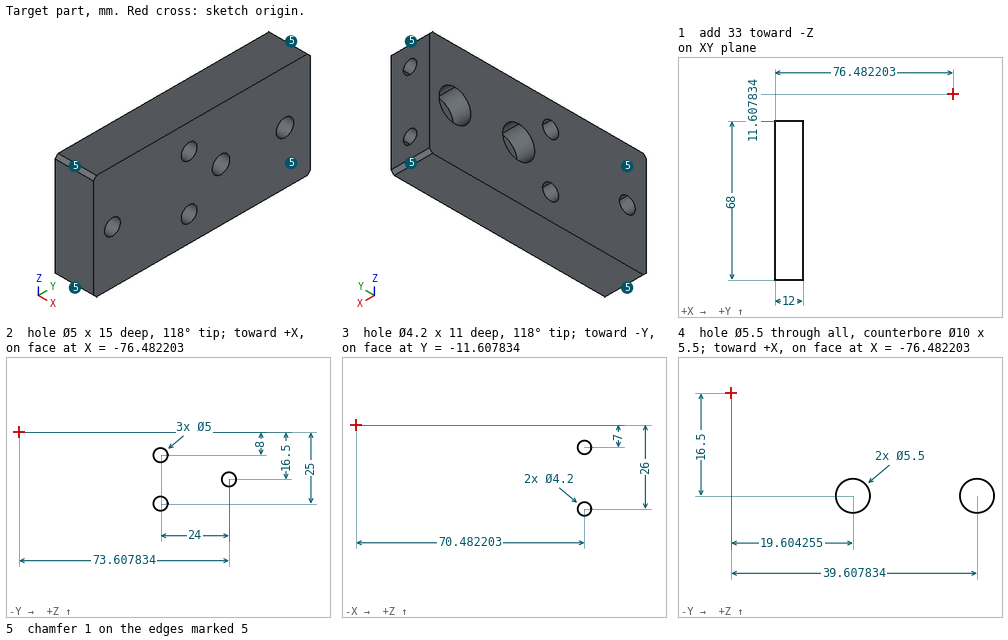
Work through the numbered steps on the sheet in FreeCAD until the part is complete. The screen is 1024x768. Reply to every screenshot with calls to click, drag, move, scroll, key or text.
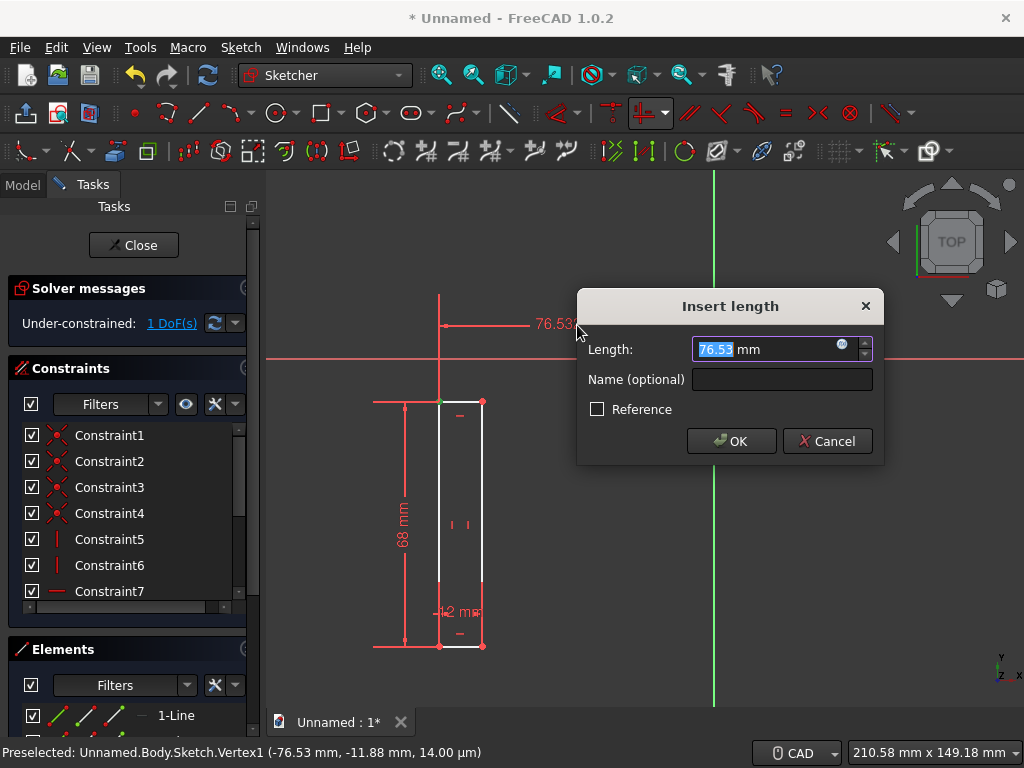
text(76.482203)
key(Return)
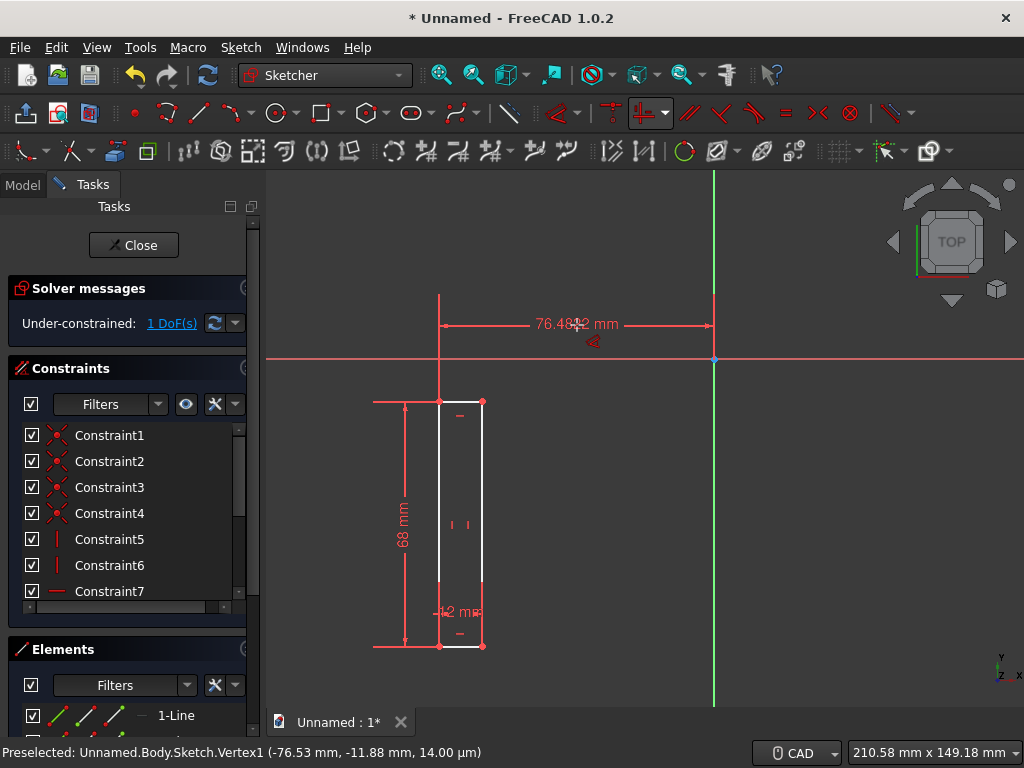
click(439, 402)
click(405, 381)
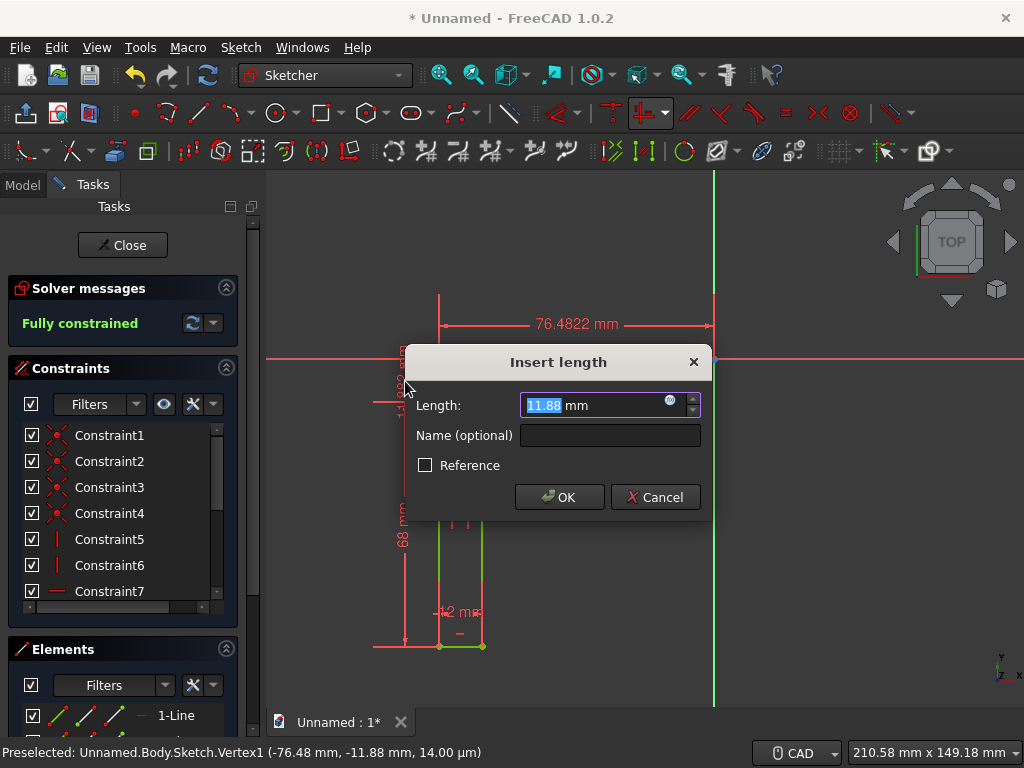
text(11.607834)
key(Return)
key(Escape)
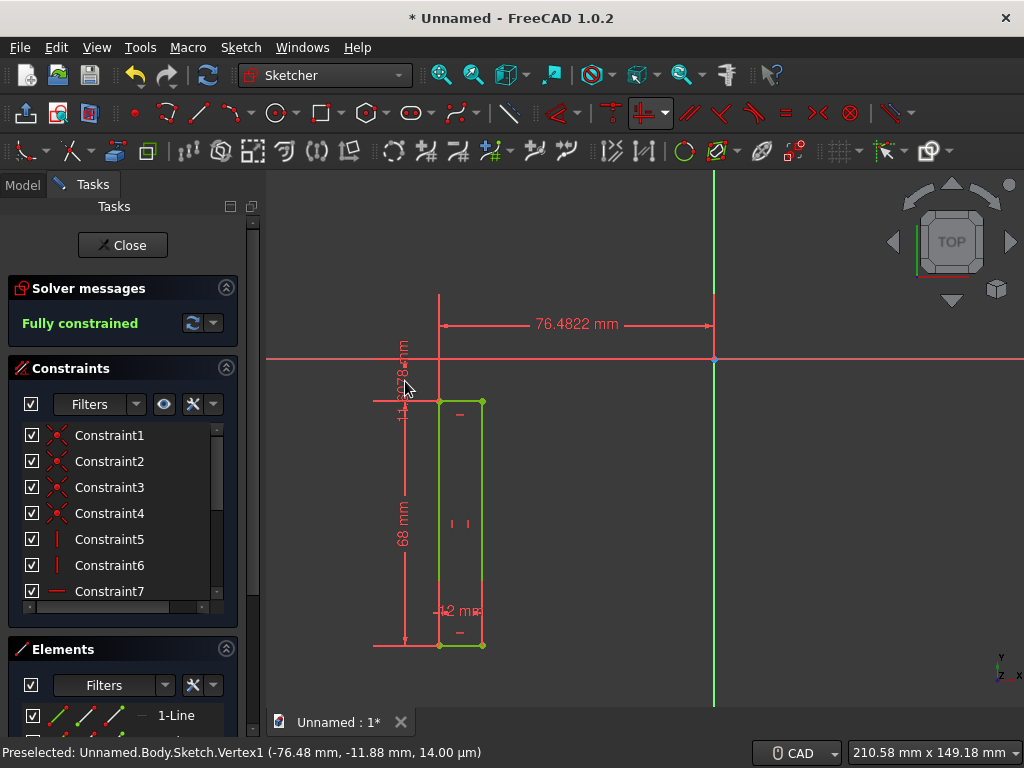
click(123, 245)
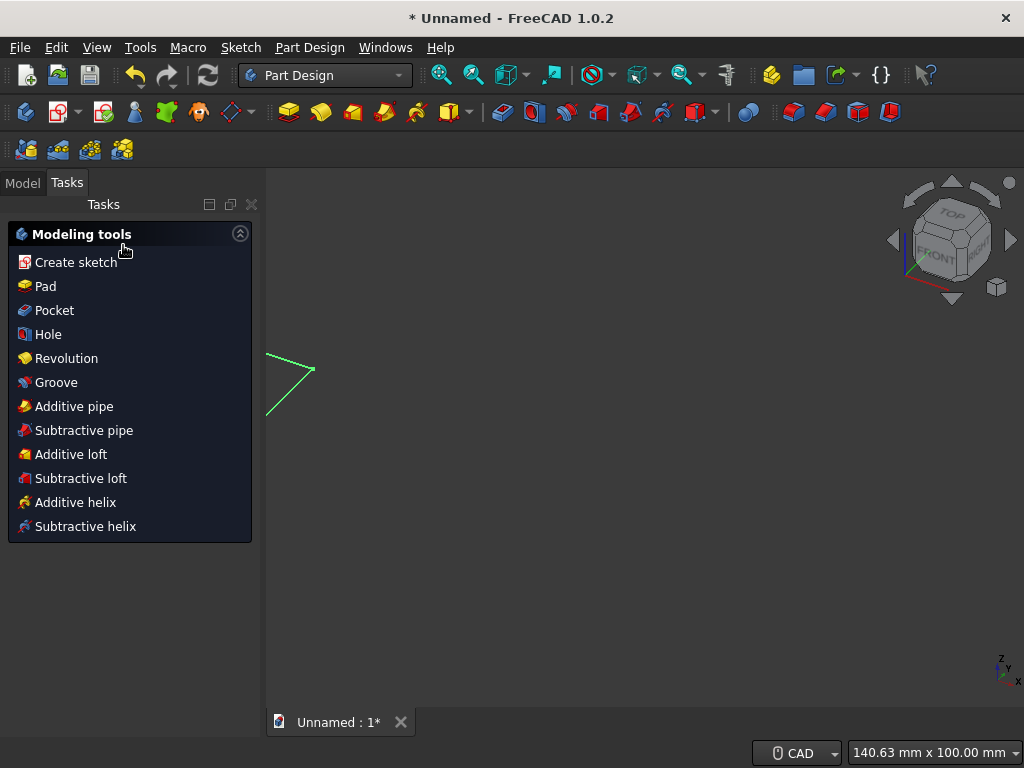
click(290, 112)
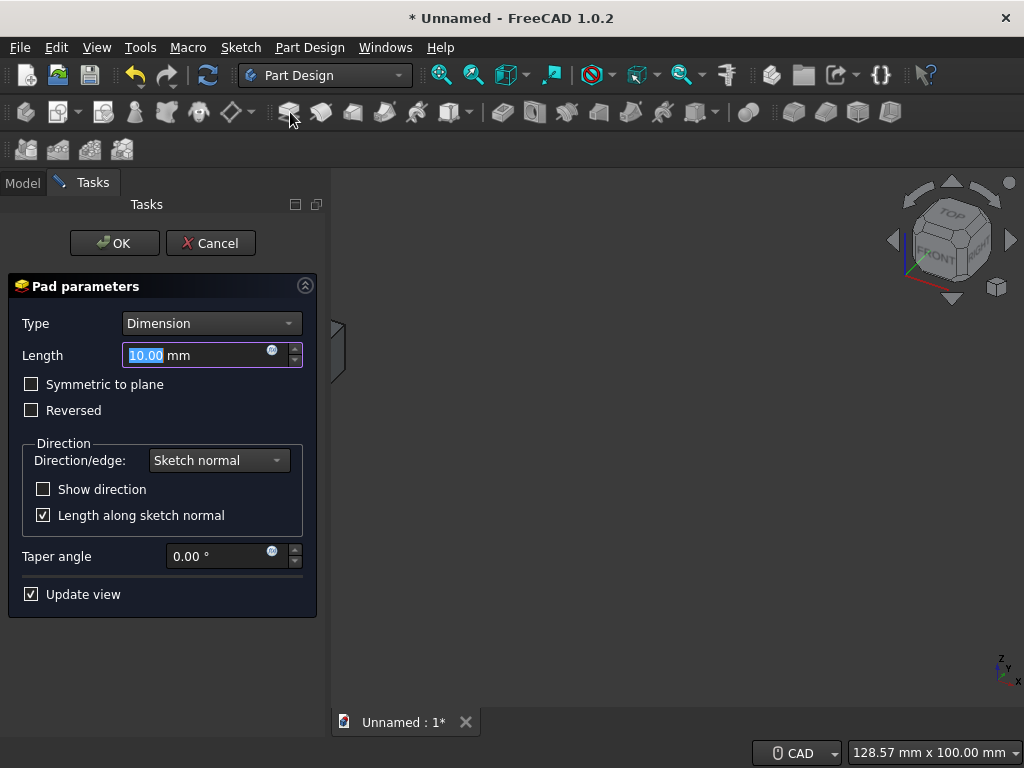
text(33)
key(Tab)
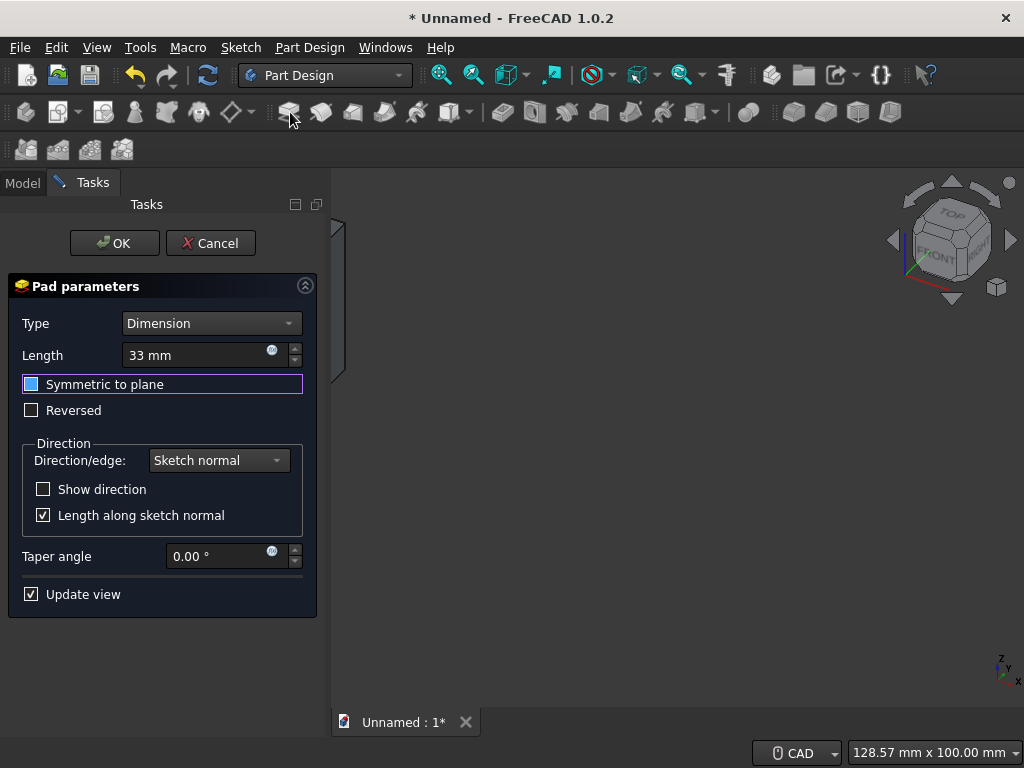
click(30, 410)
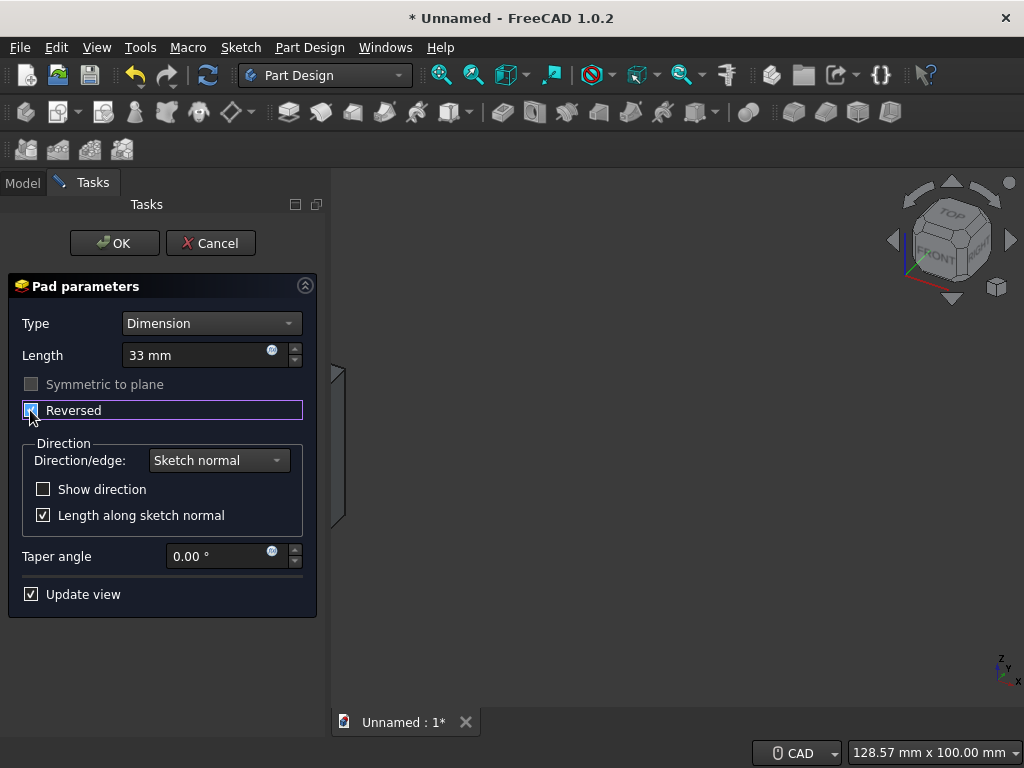
click(115, 243)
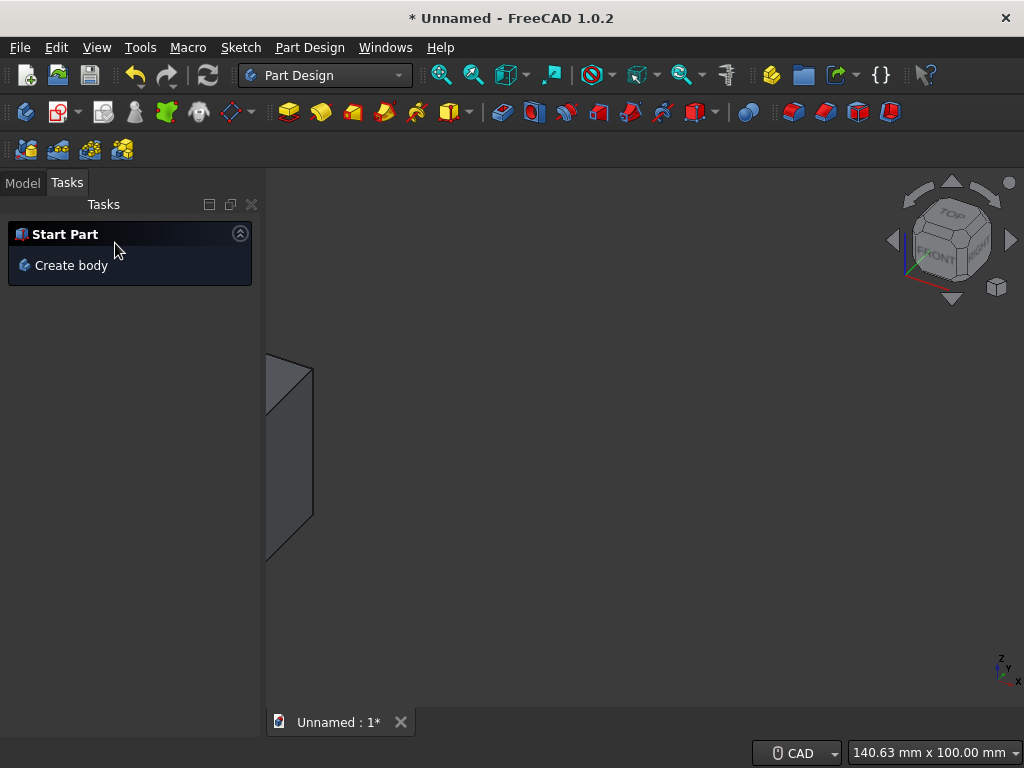
key(v)
key(f)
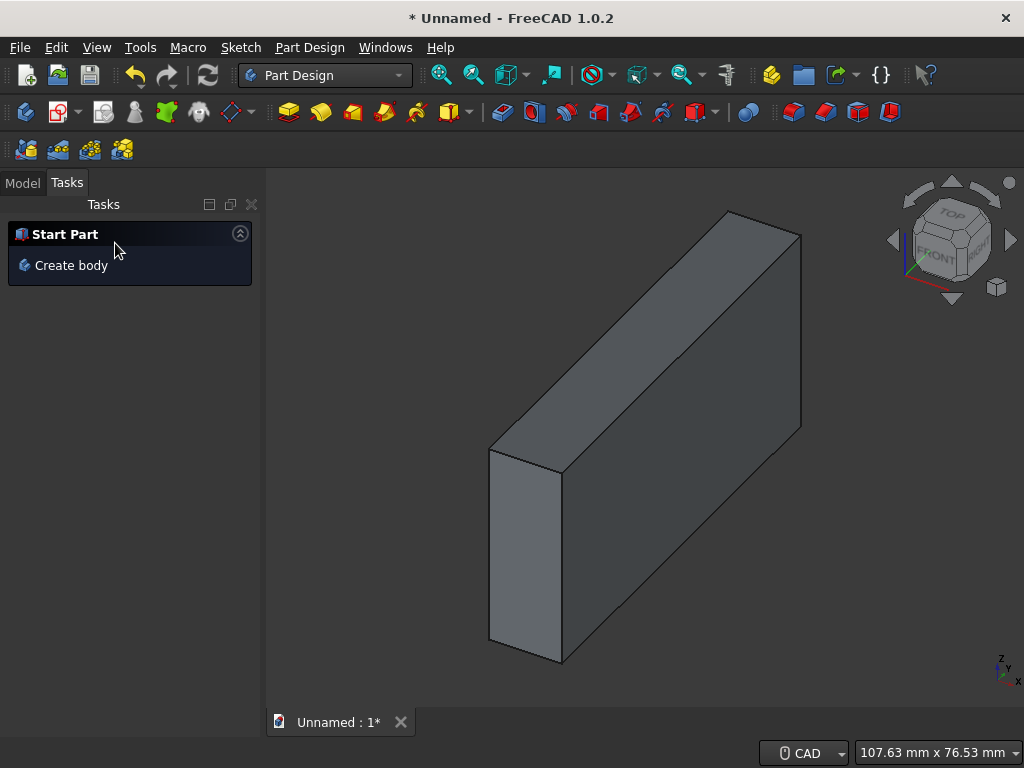
key(6)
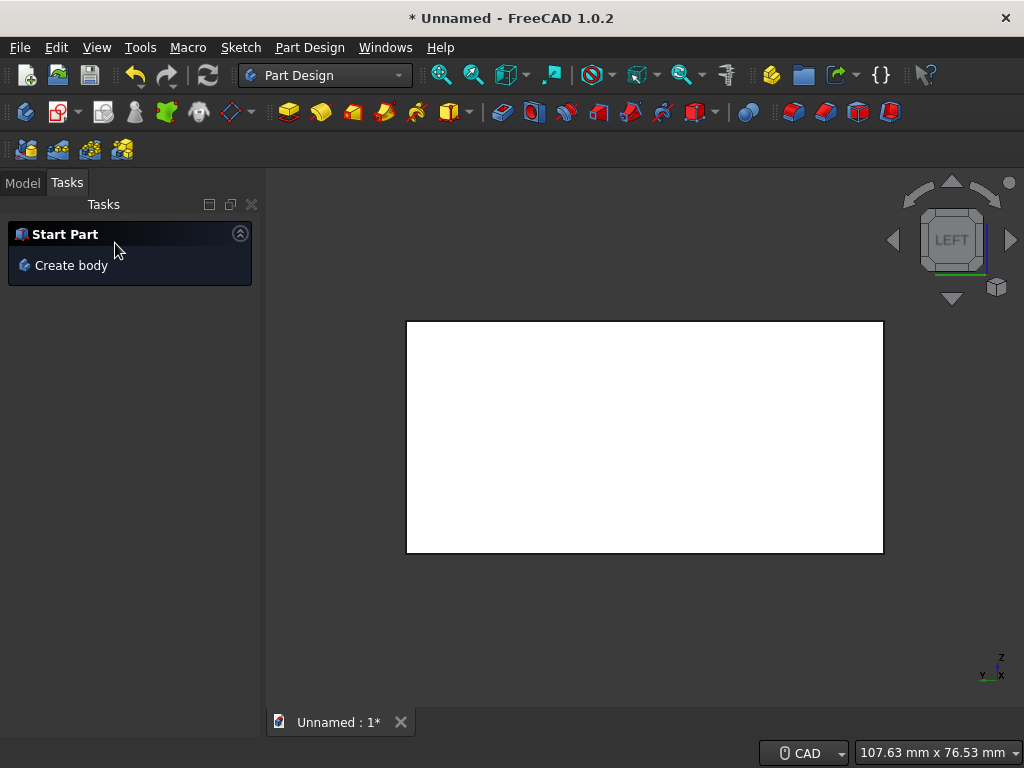
click(577, 436)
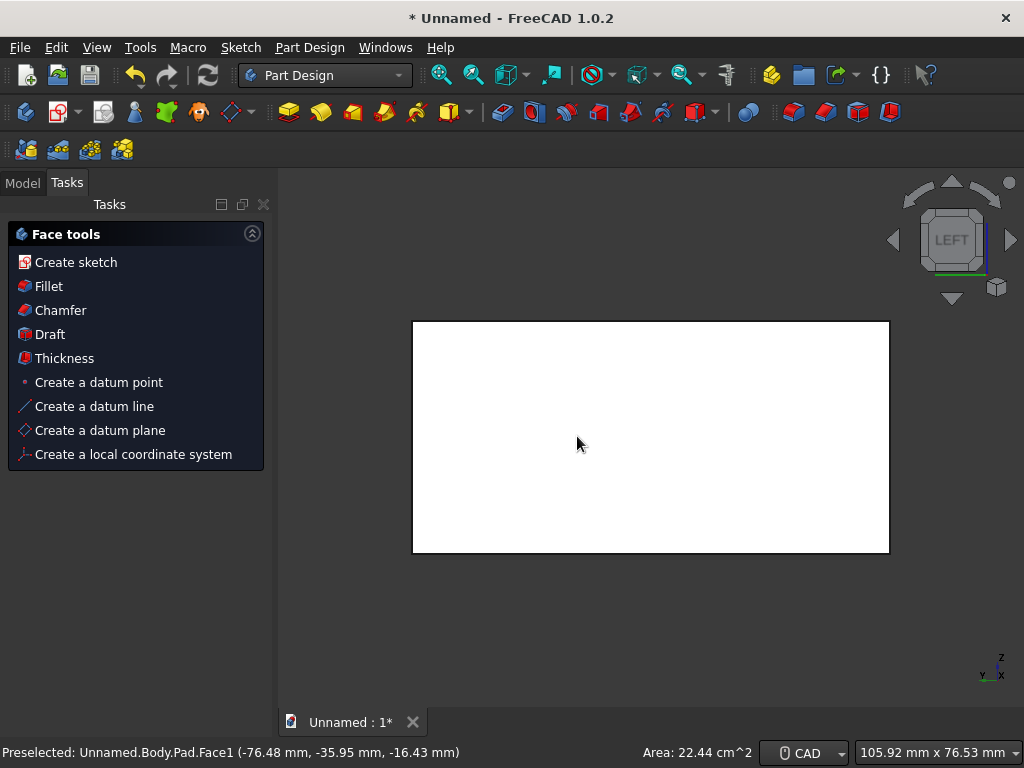
click(58, 112)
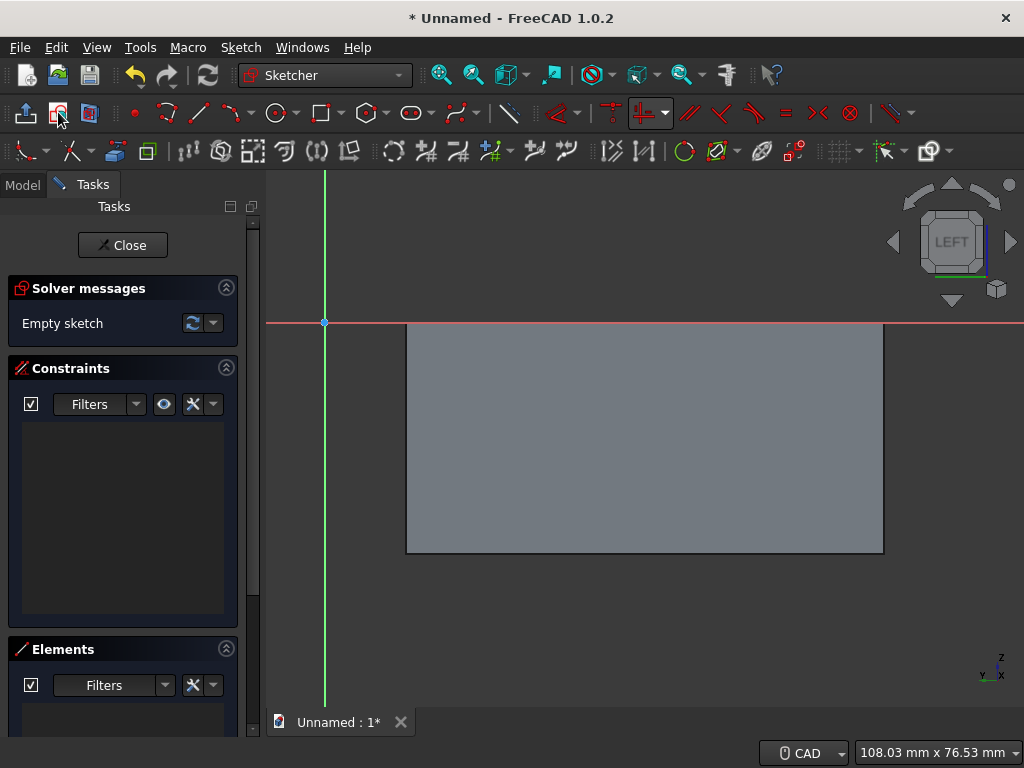
scroll(576, 438, down, 5)